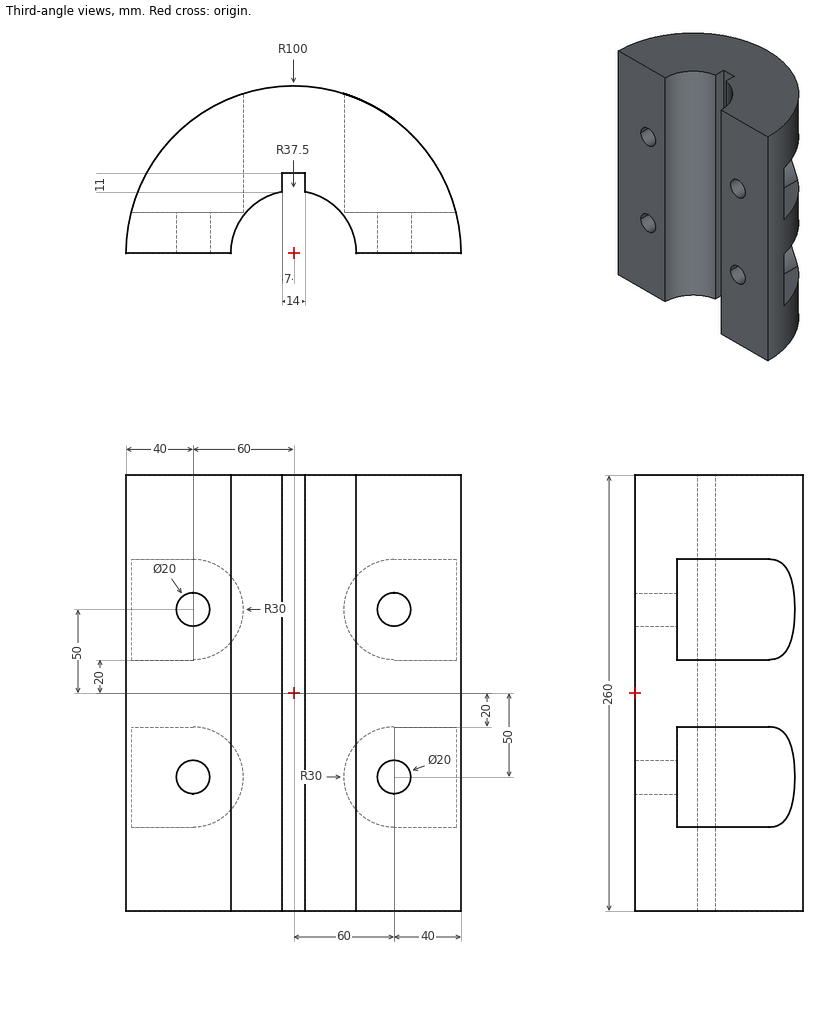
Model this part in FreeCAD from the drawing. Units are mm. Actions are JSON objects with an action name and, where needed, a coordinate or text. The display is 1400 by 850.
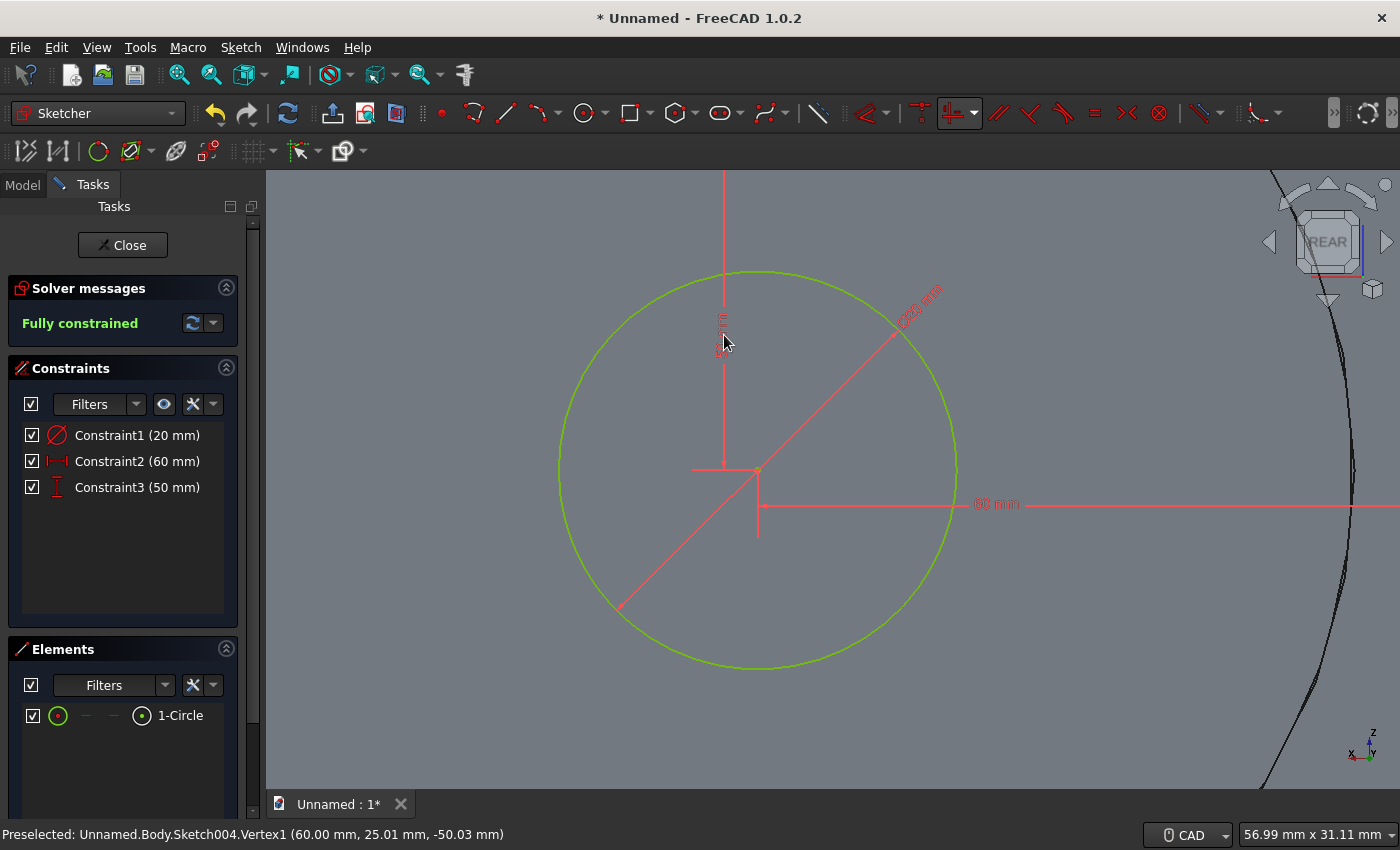
{"action": "left_click", "coordinate": [123, 245]}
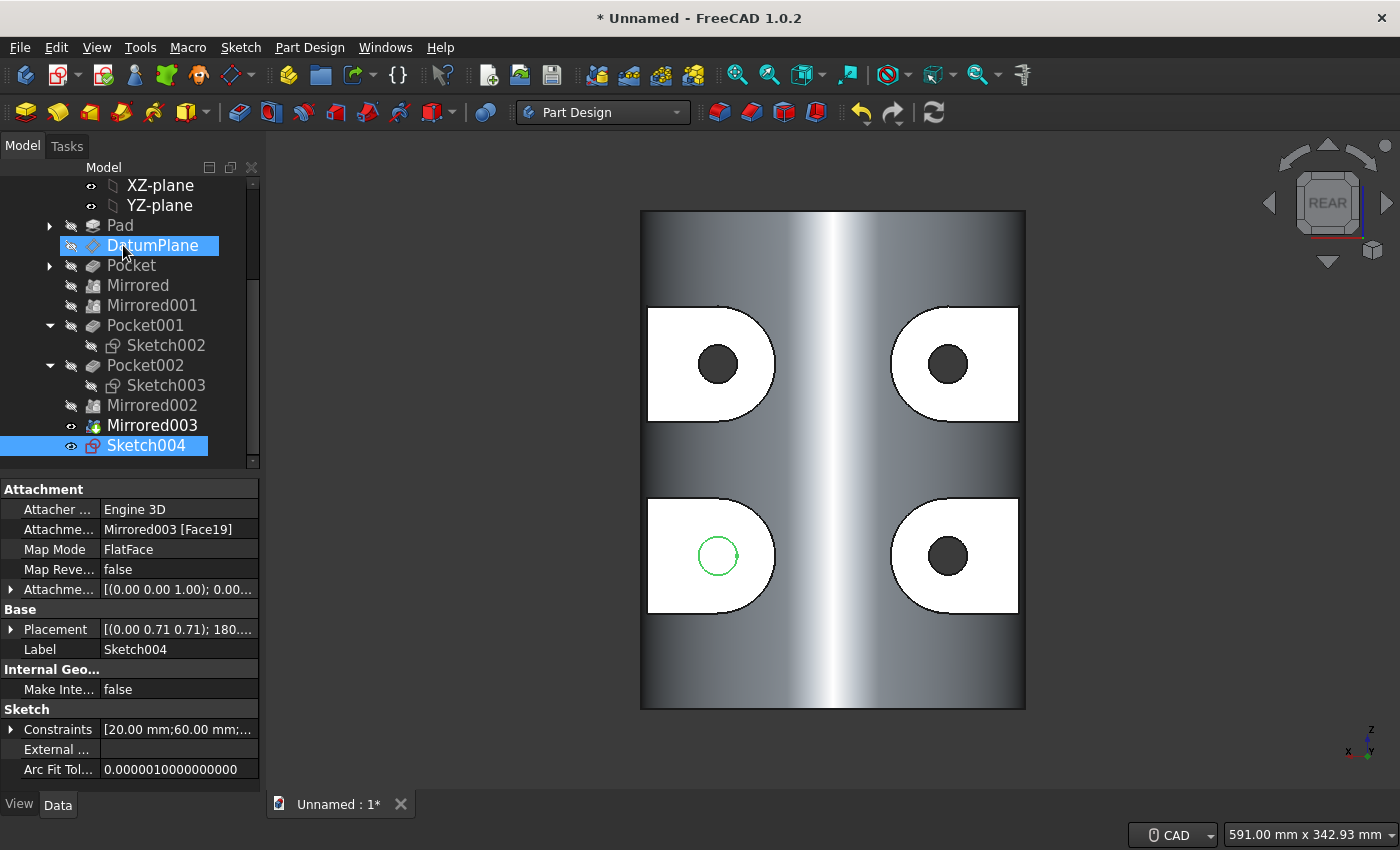
{"action": "left_click", "coordinate": [240, 112]}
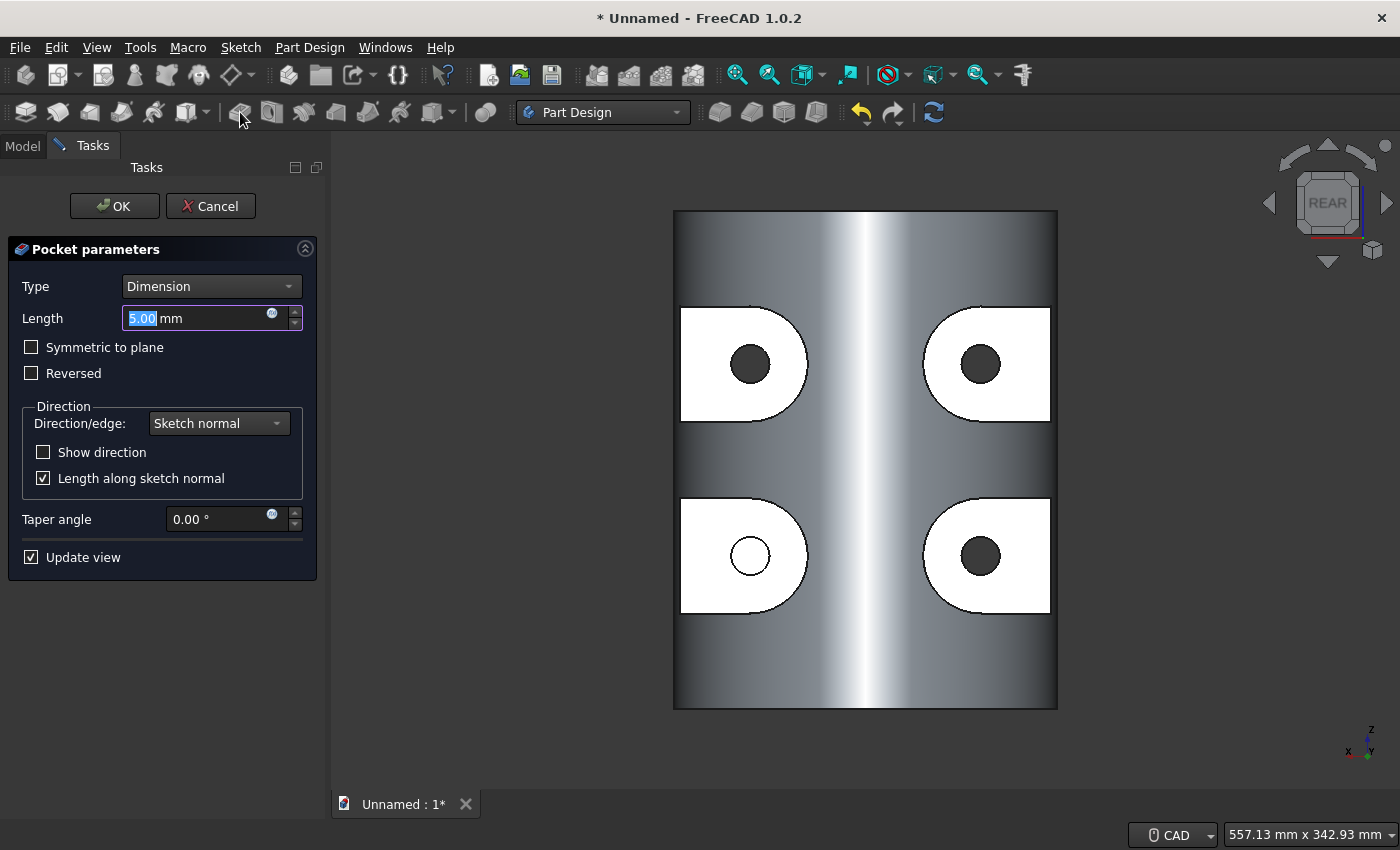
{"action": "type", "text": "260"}
{"action": "key", "text": "Tab"}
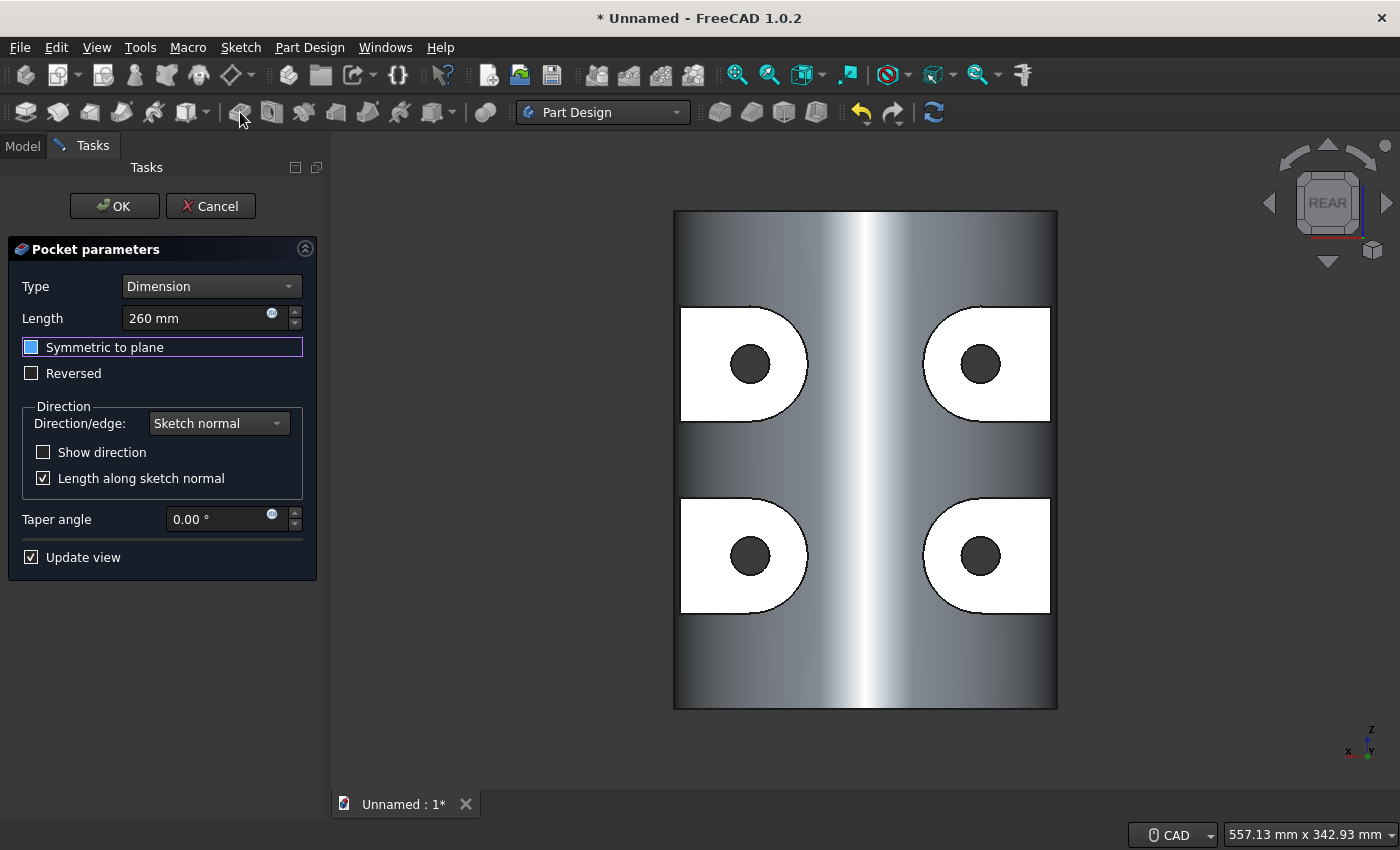
{"action": "left_click", "coordinate": [115, 206]}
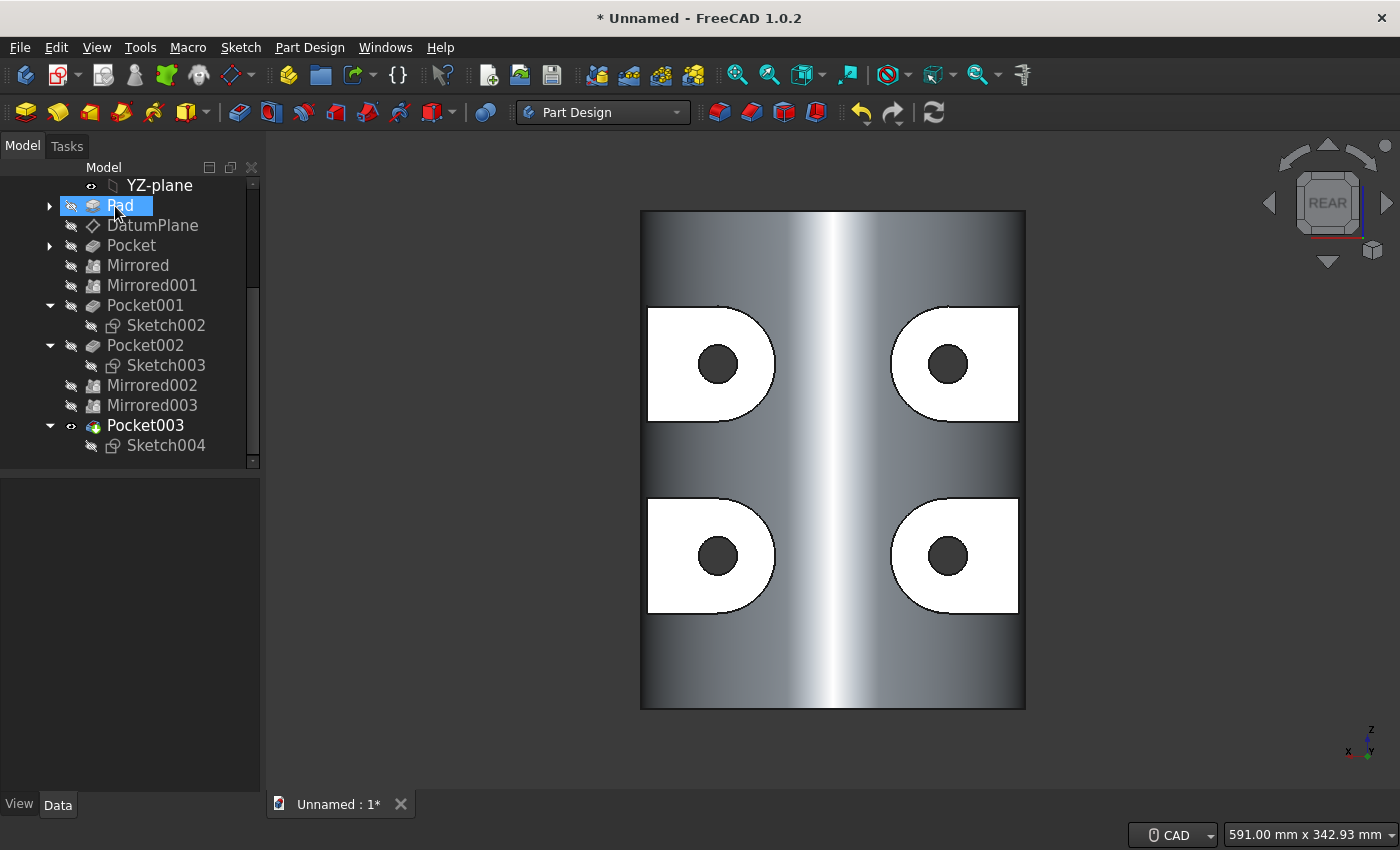
{"action": "key", "text": "5"}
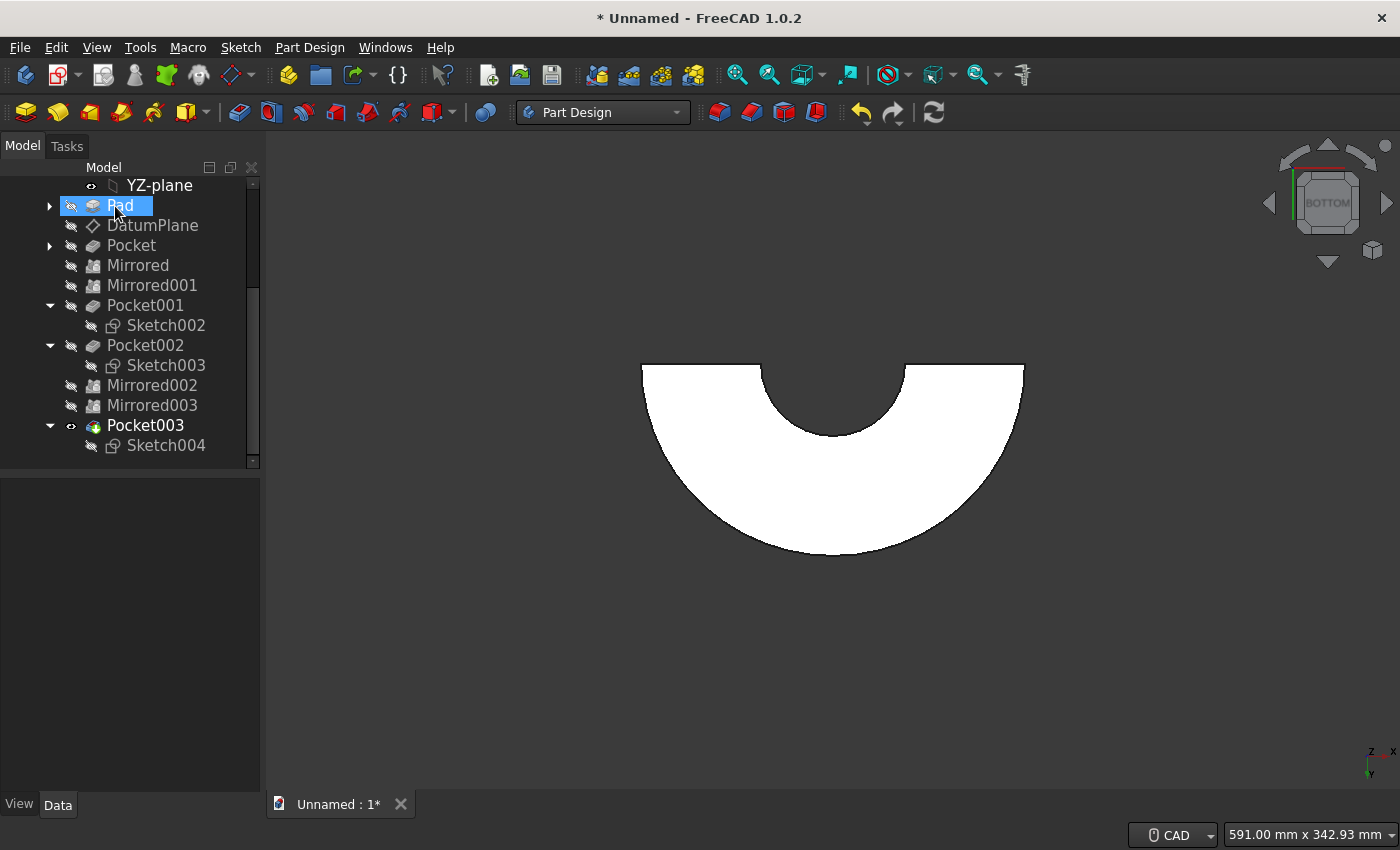
{"action": "left_click", "coordinate": [738, 76]}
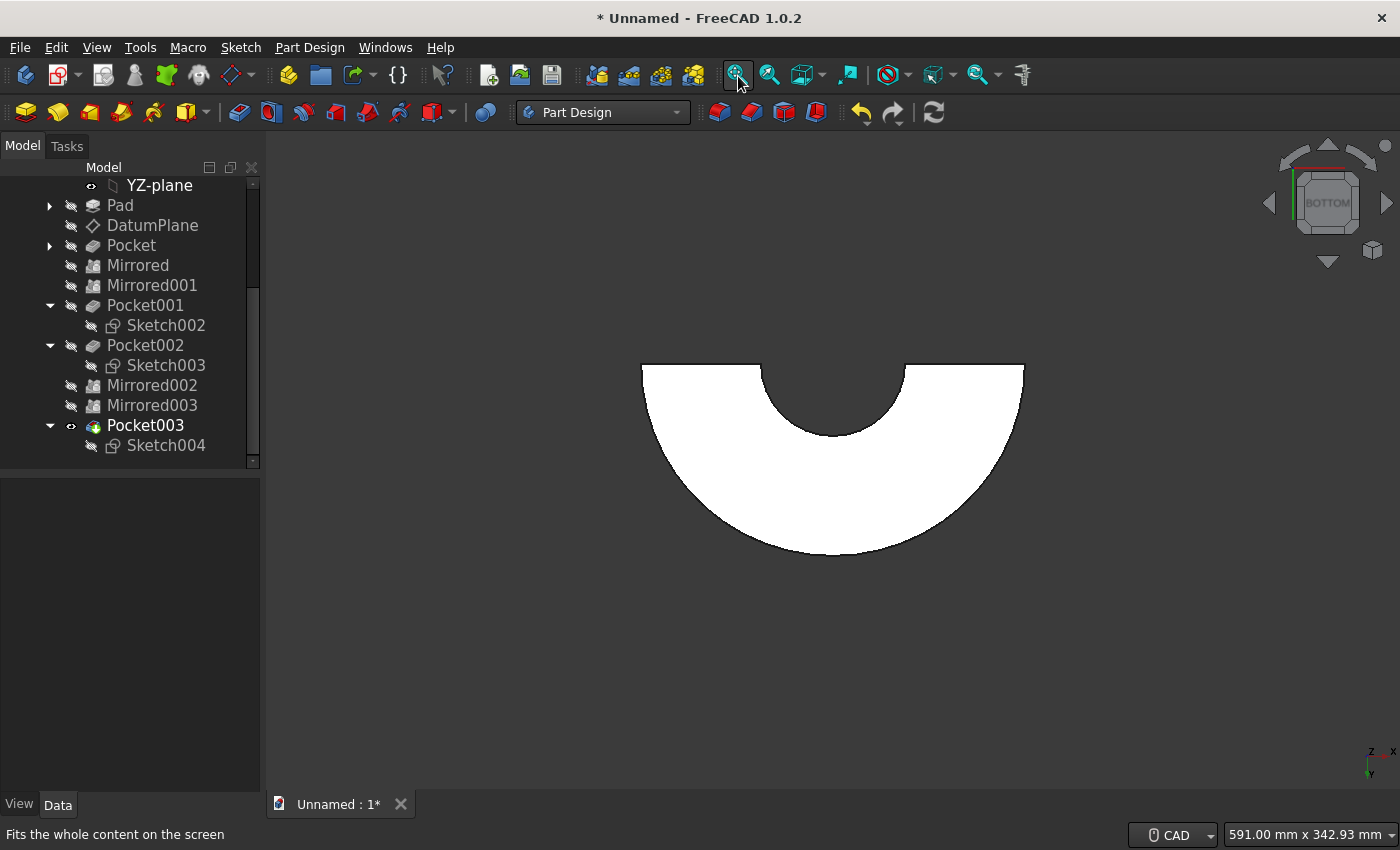
{"action": "left_click", "coordinate": [723, 432]}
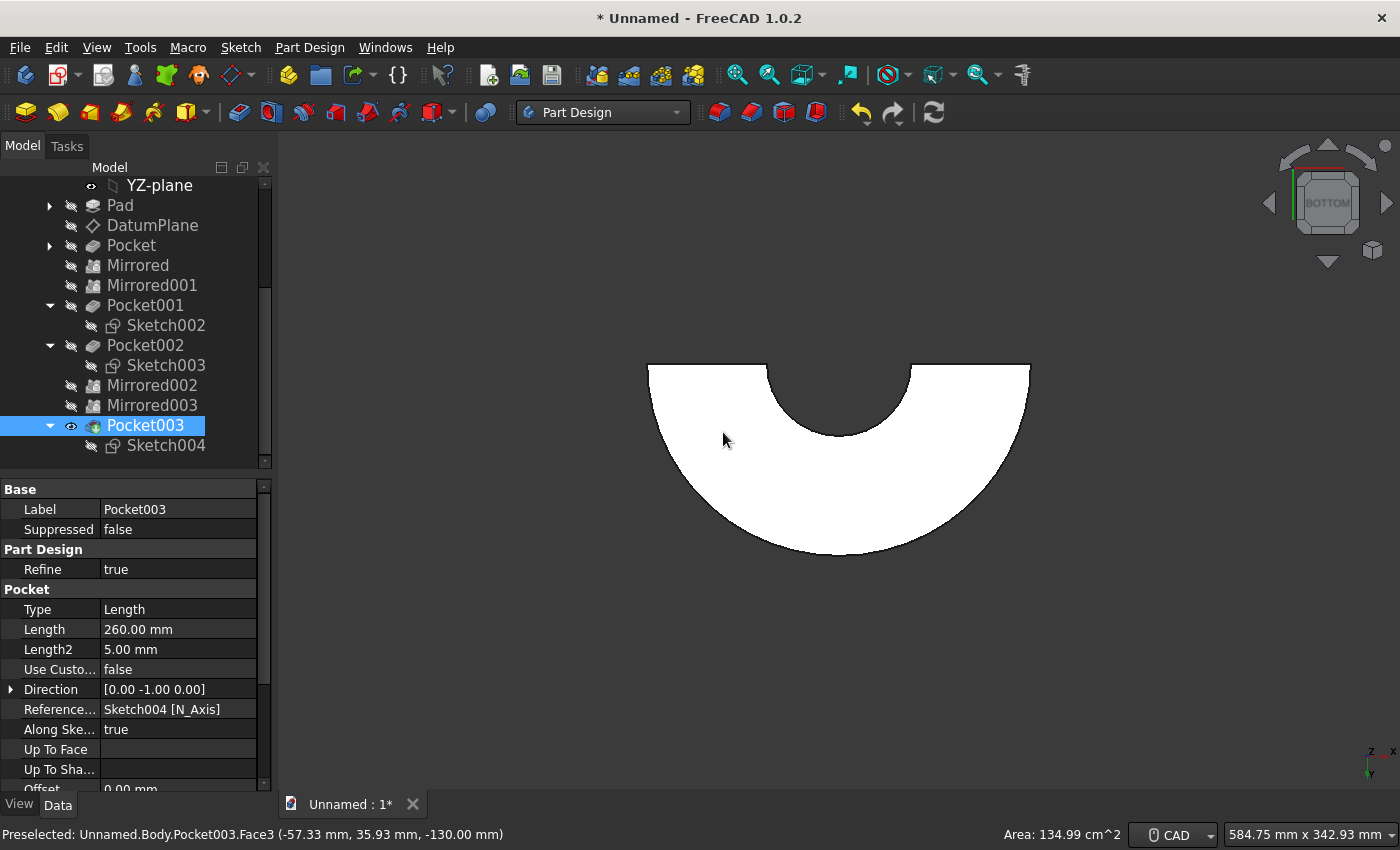
{"action": "left_click", "coordinate": [58, 76]}